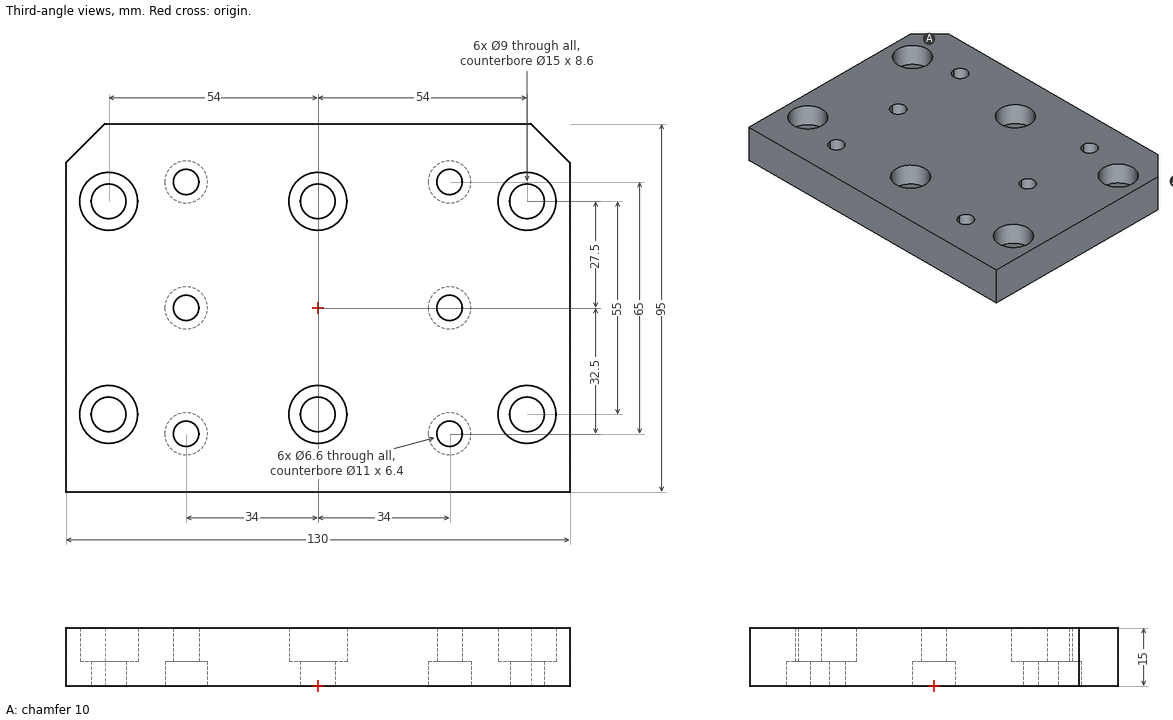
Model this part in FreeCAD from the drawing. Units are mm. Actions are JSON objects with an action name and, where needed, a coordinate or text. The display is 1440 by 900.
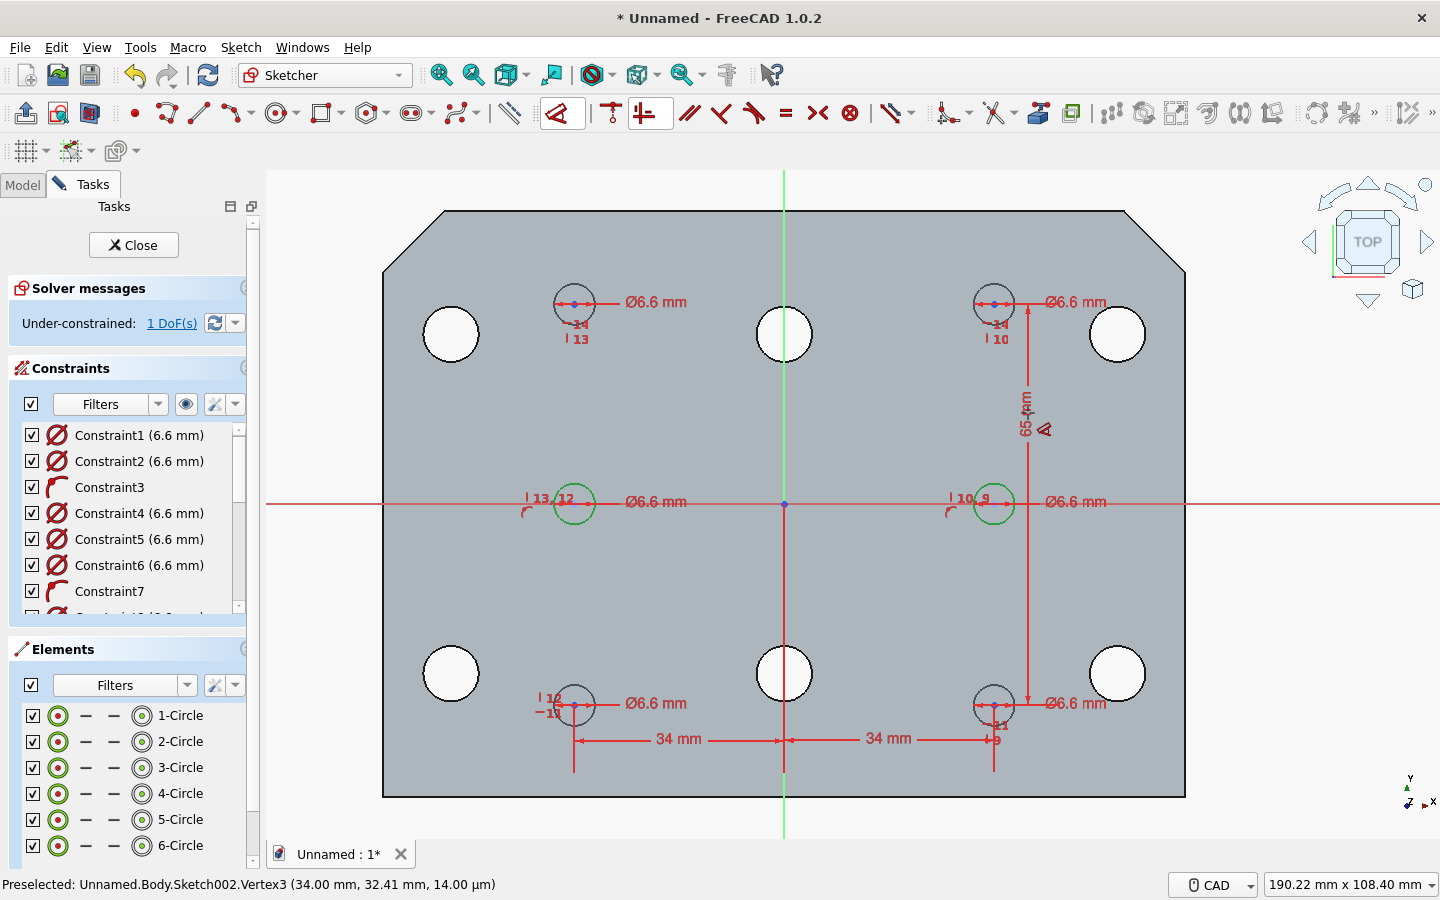
{"action": "left_click", "coordinate": [994, 705]}
{"action": "left_click", "coordinate": [1028, 605]}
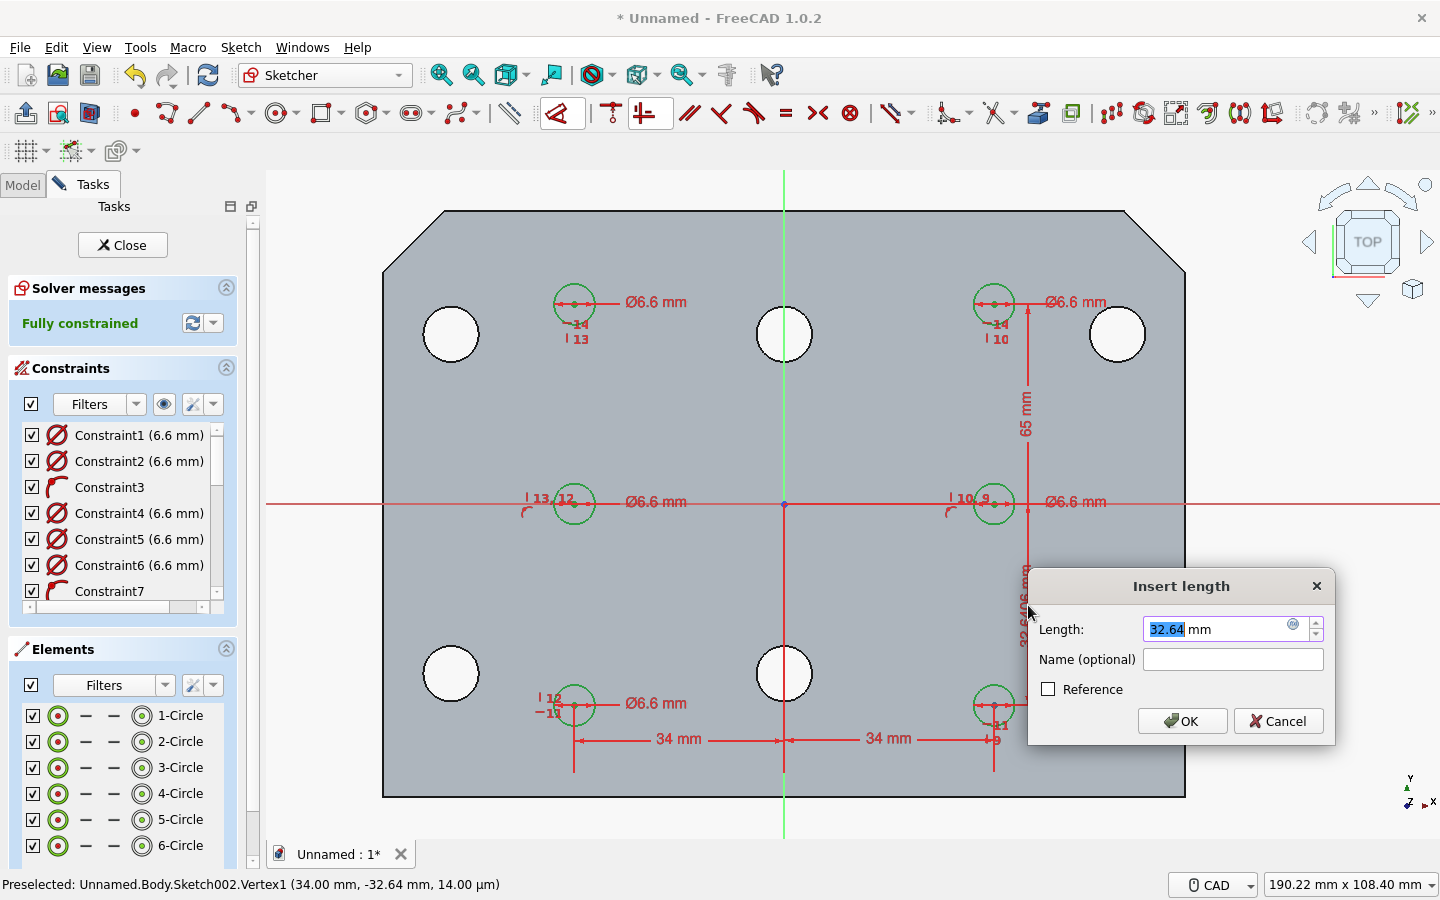
{"action": "type", "text": "32.5"}
{"action": "key", "text": "Return"}
{"action": "key", "text": "Escape"}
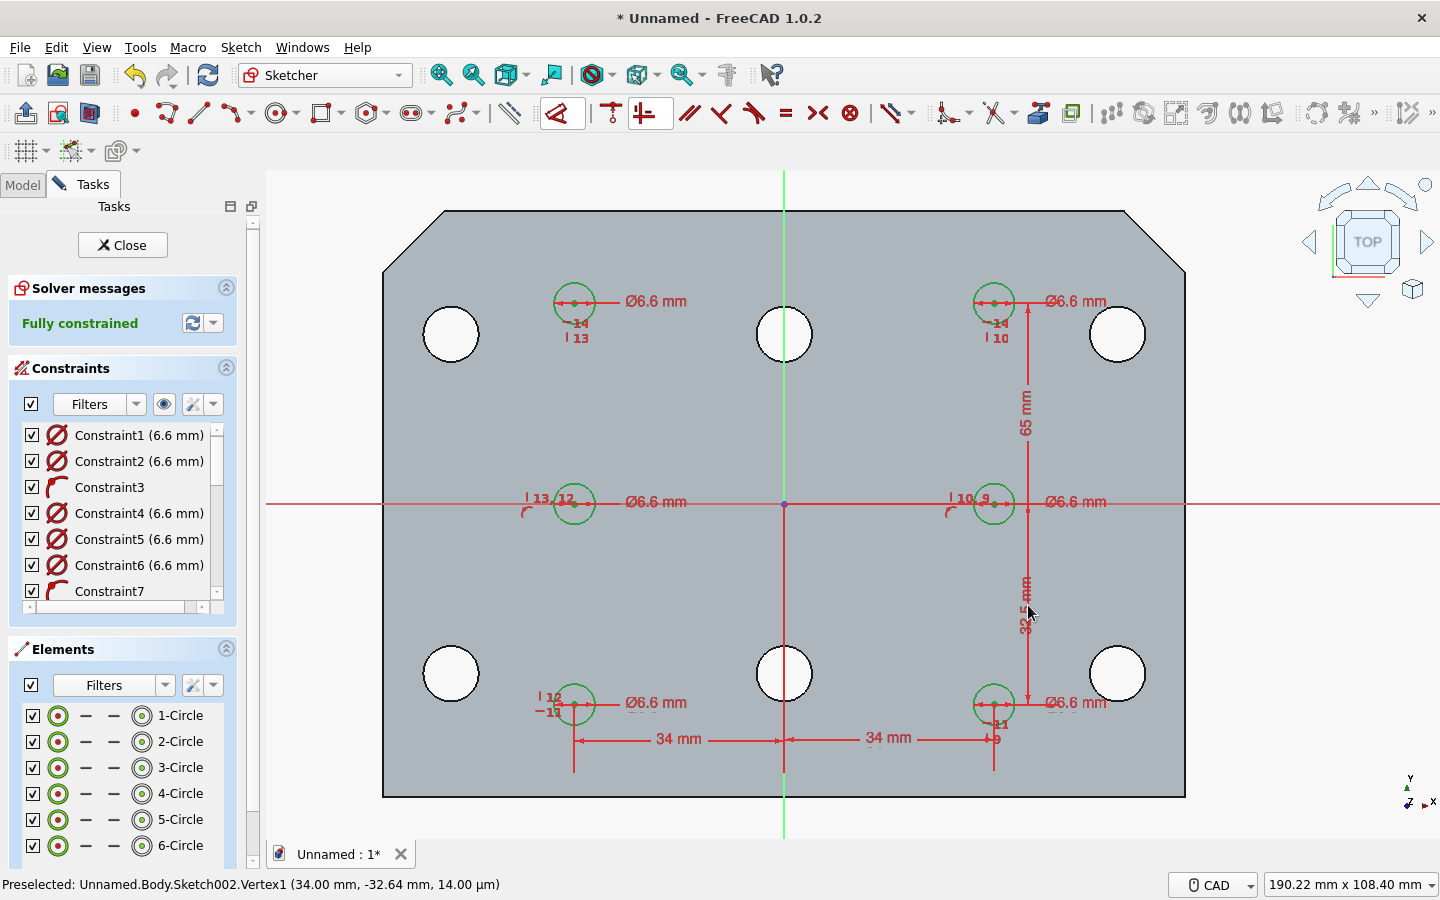
{"action": "left_click", "coordinate": [123, 245]}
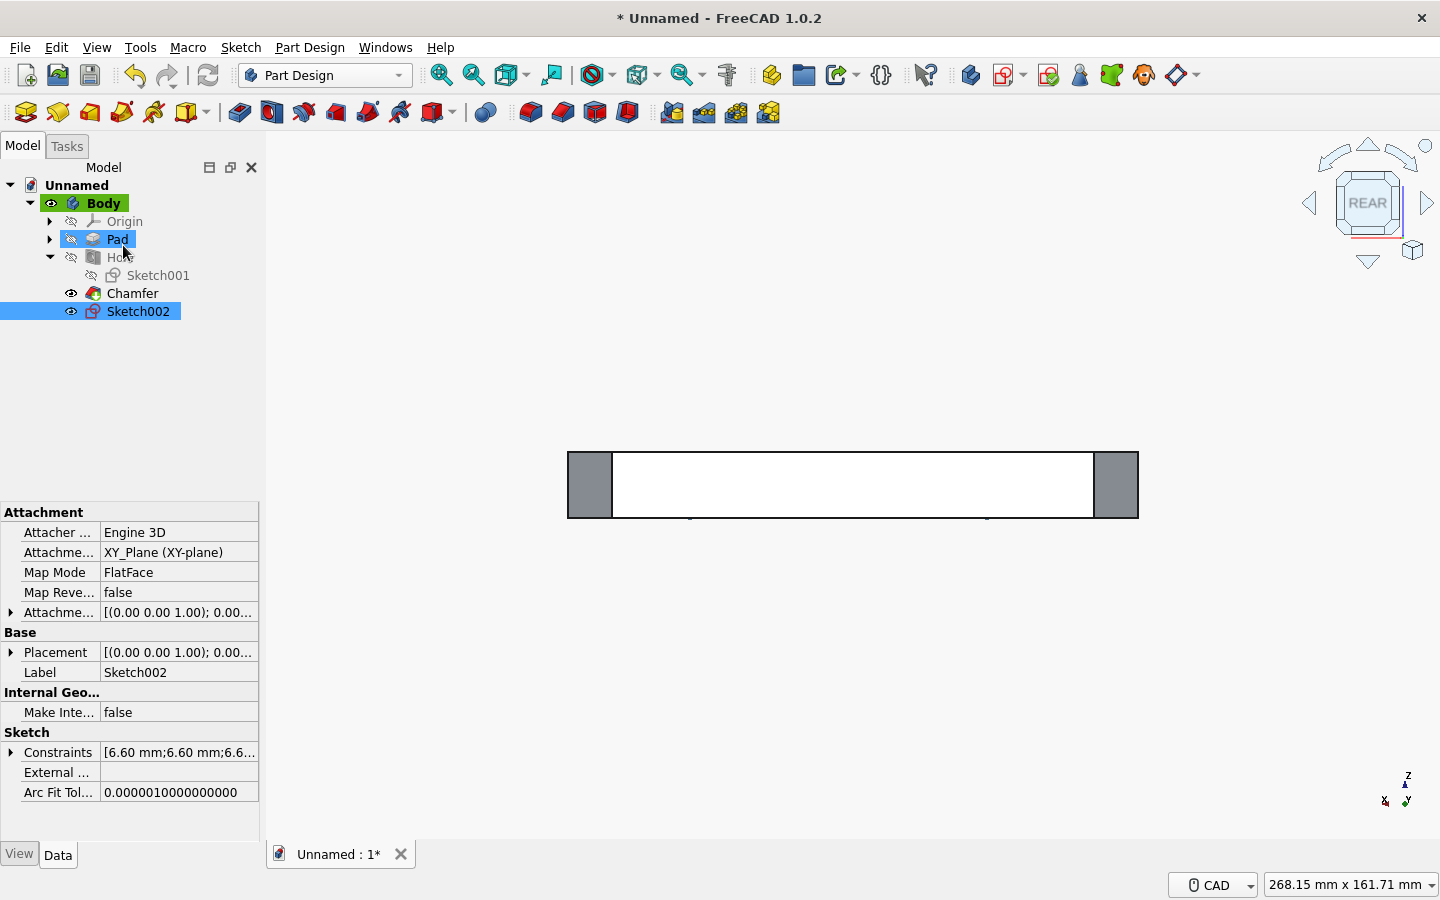
{"action": "left_click", "coordinate": [272, 112]}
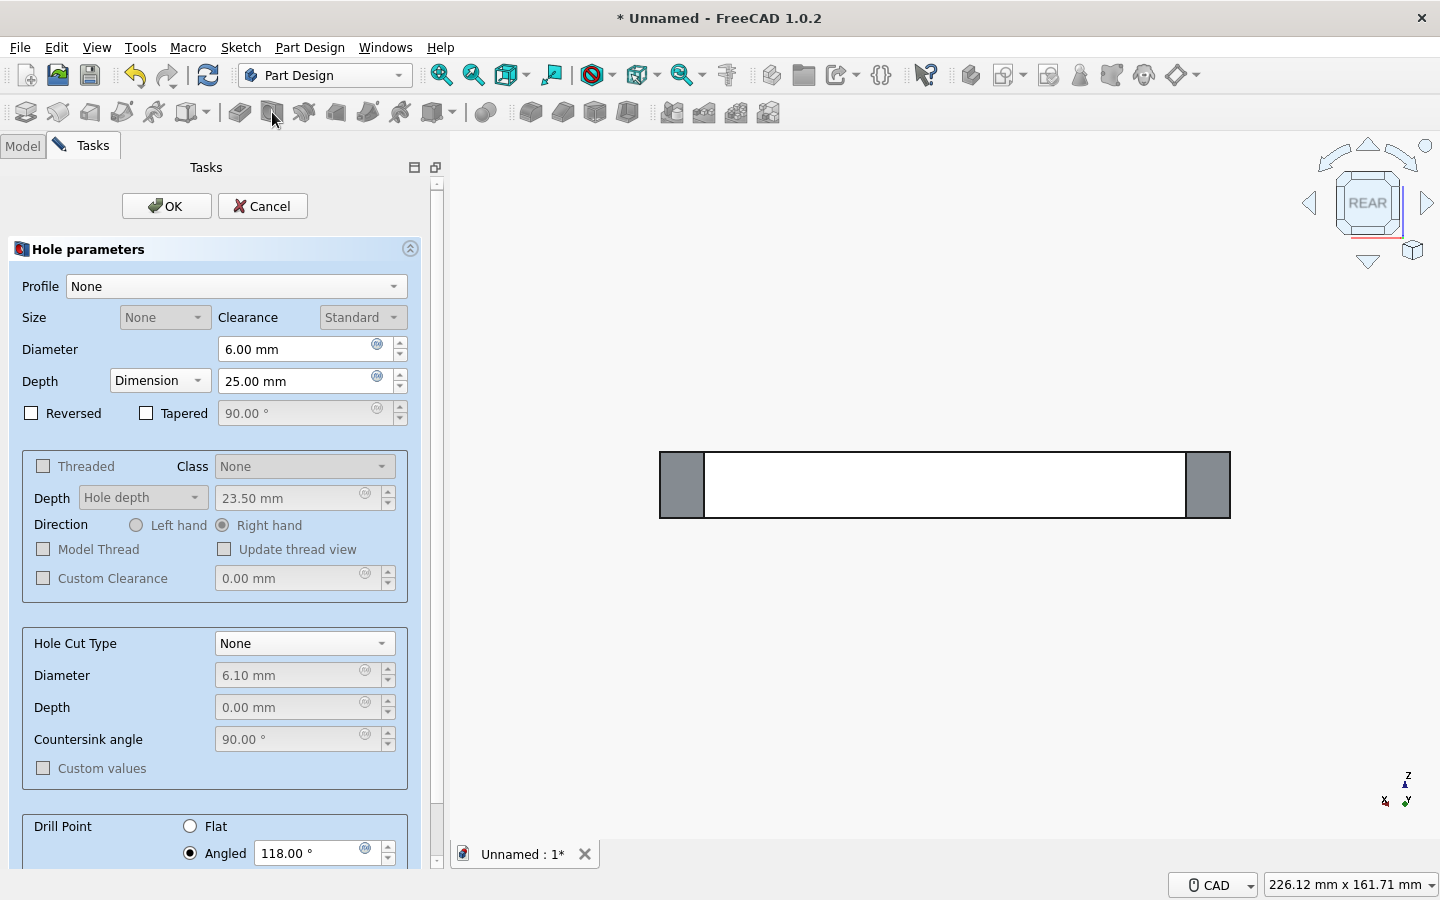
{"action": "triple_click", "coordinate": [305, 349]}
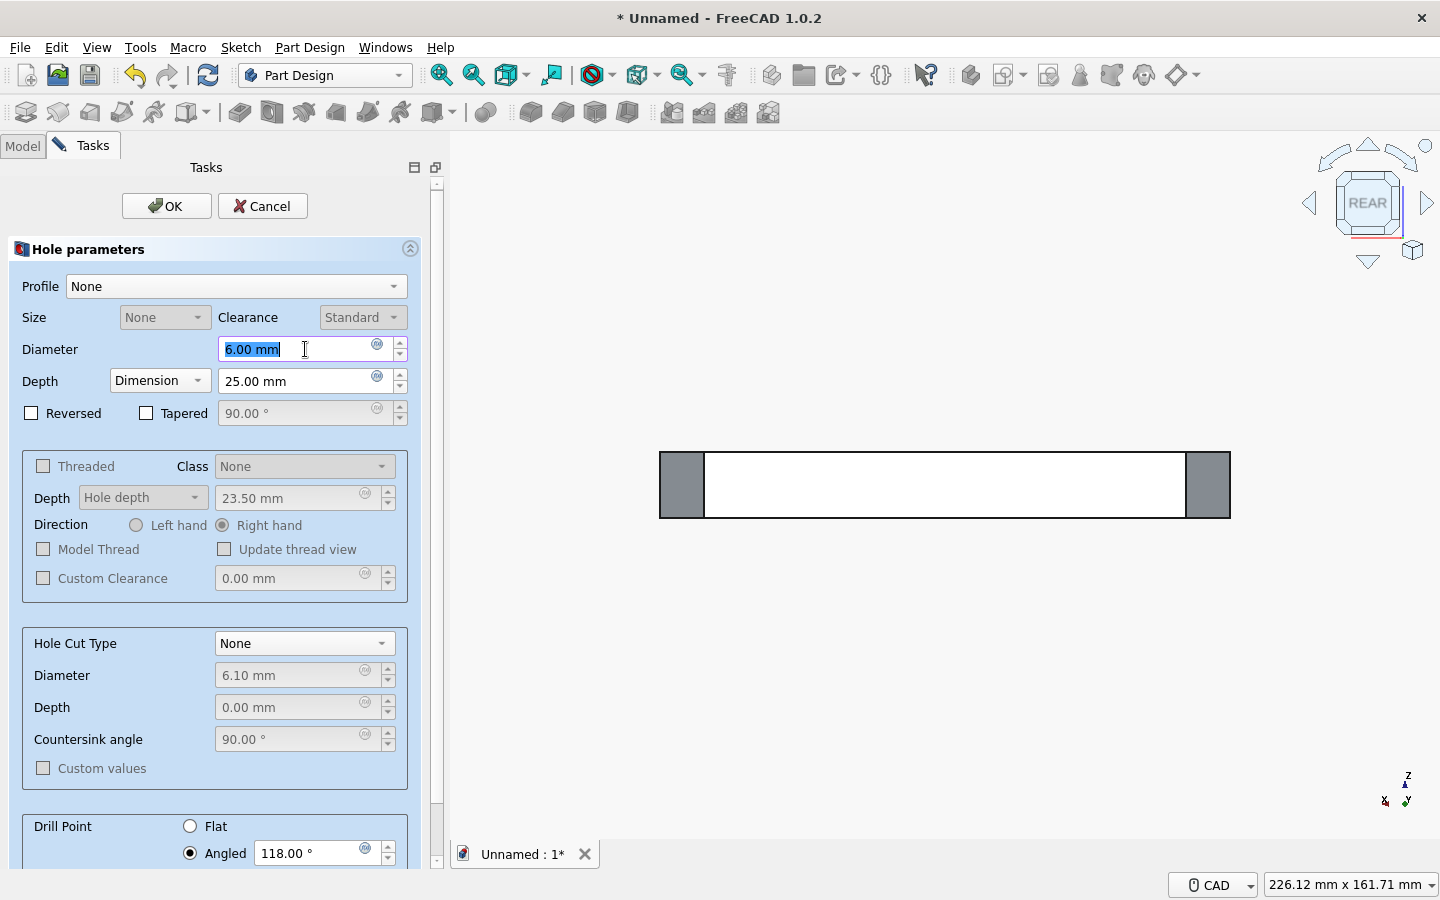
{"action": "type", "text": "6.6"}
{"action": "key", "text": "Tab"}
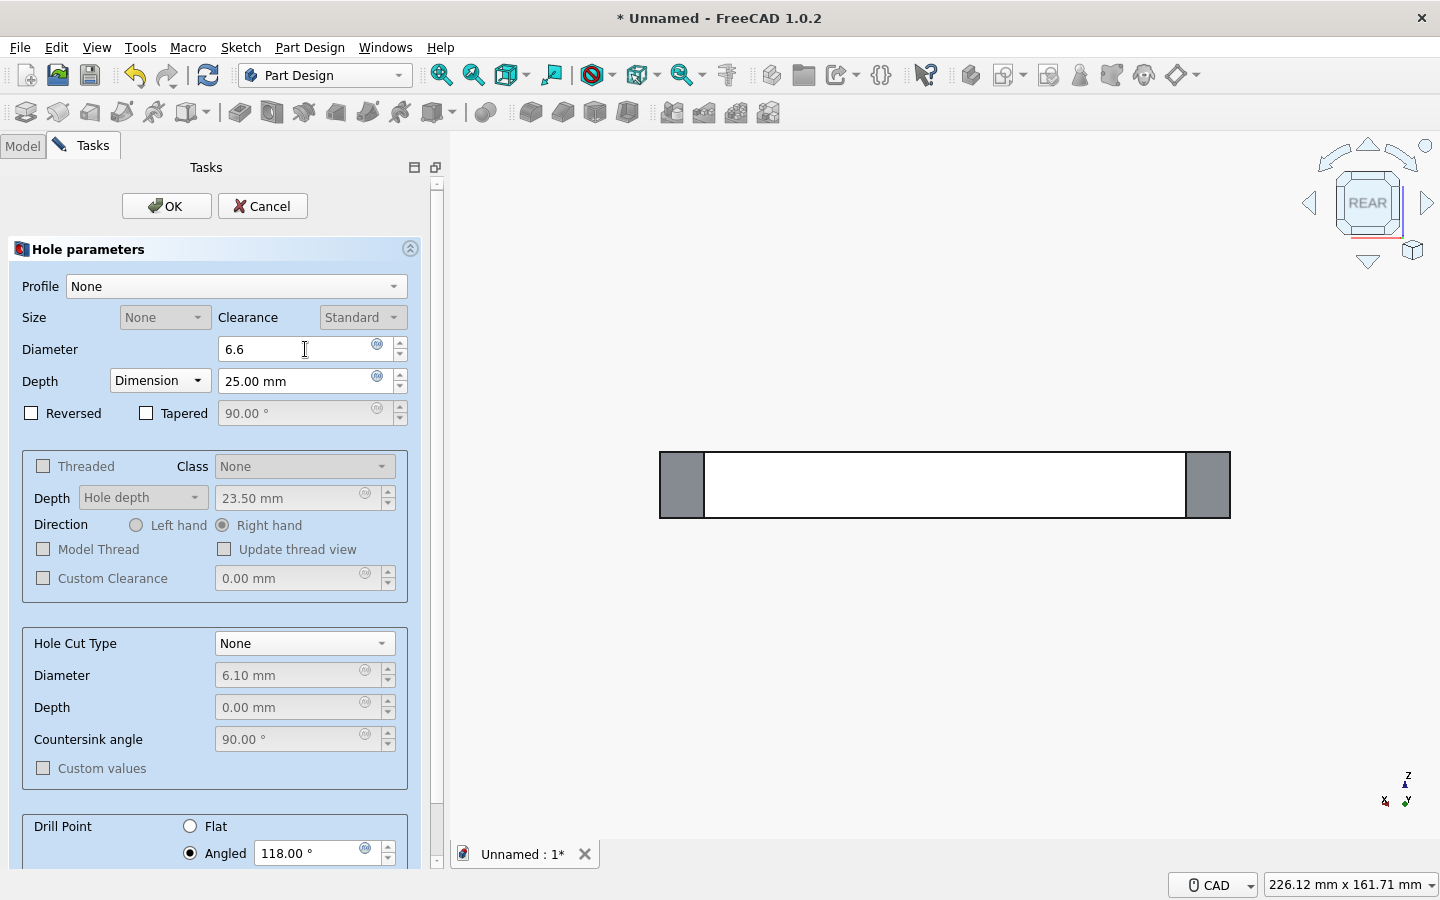
{"action": "left_click", "coordinate": [161, 380]}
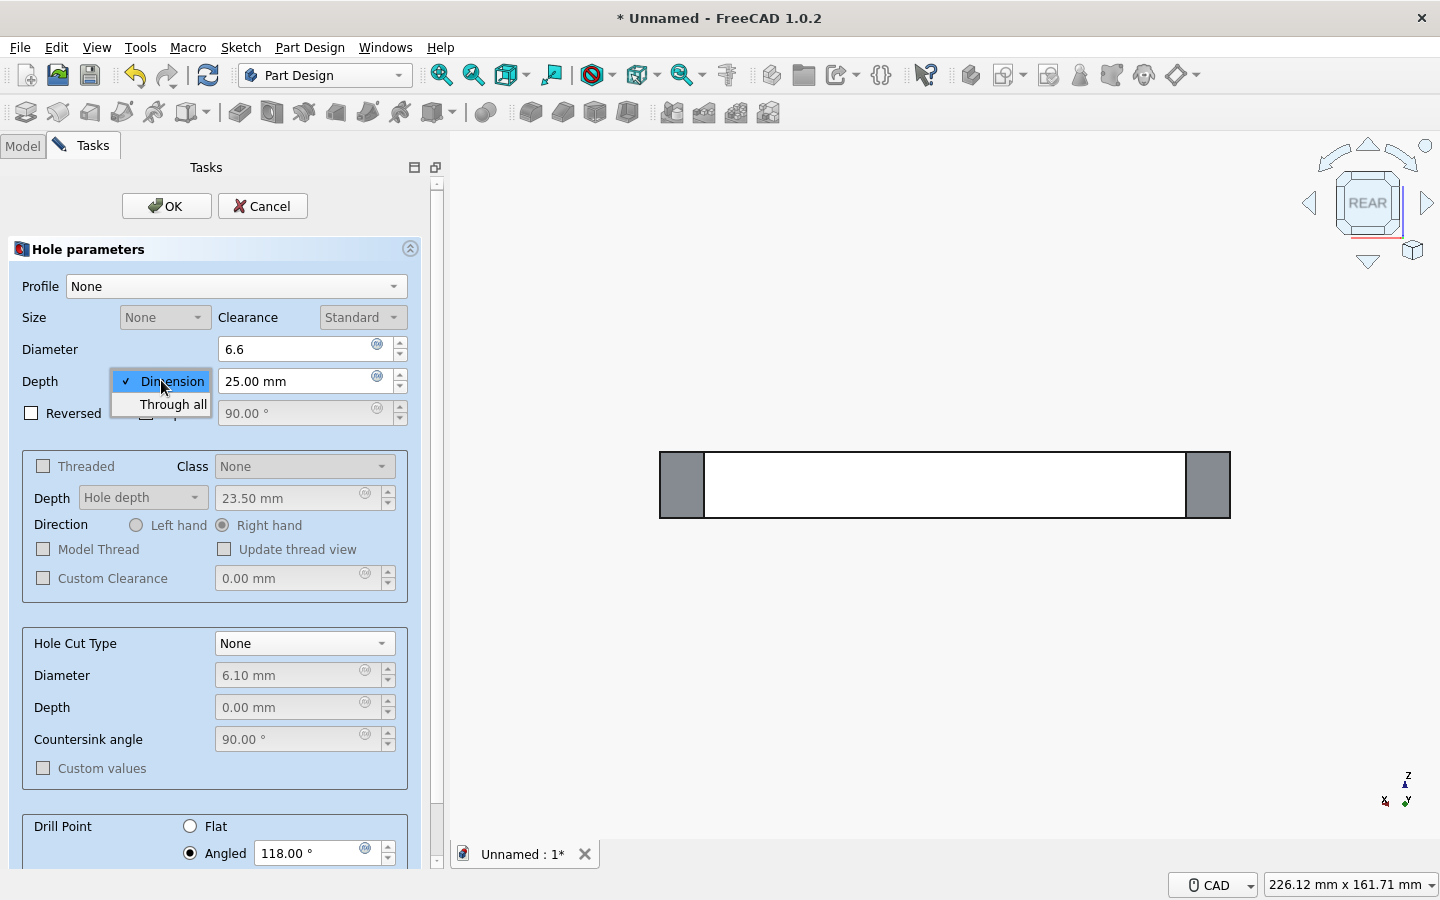
{"action": "left_click", "coordinate": [160, 404]}